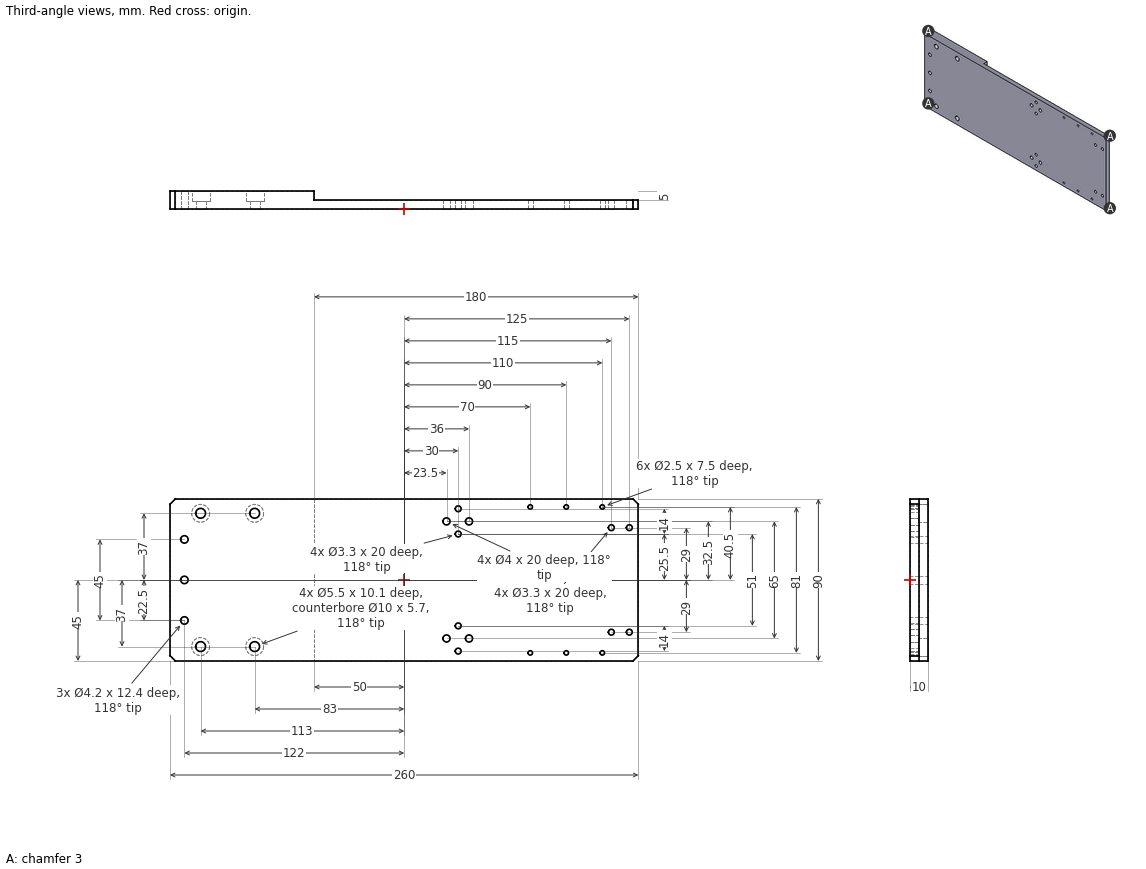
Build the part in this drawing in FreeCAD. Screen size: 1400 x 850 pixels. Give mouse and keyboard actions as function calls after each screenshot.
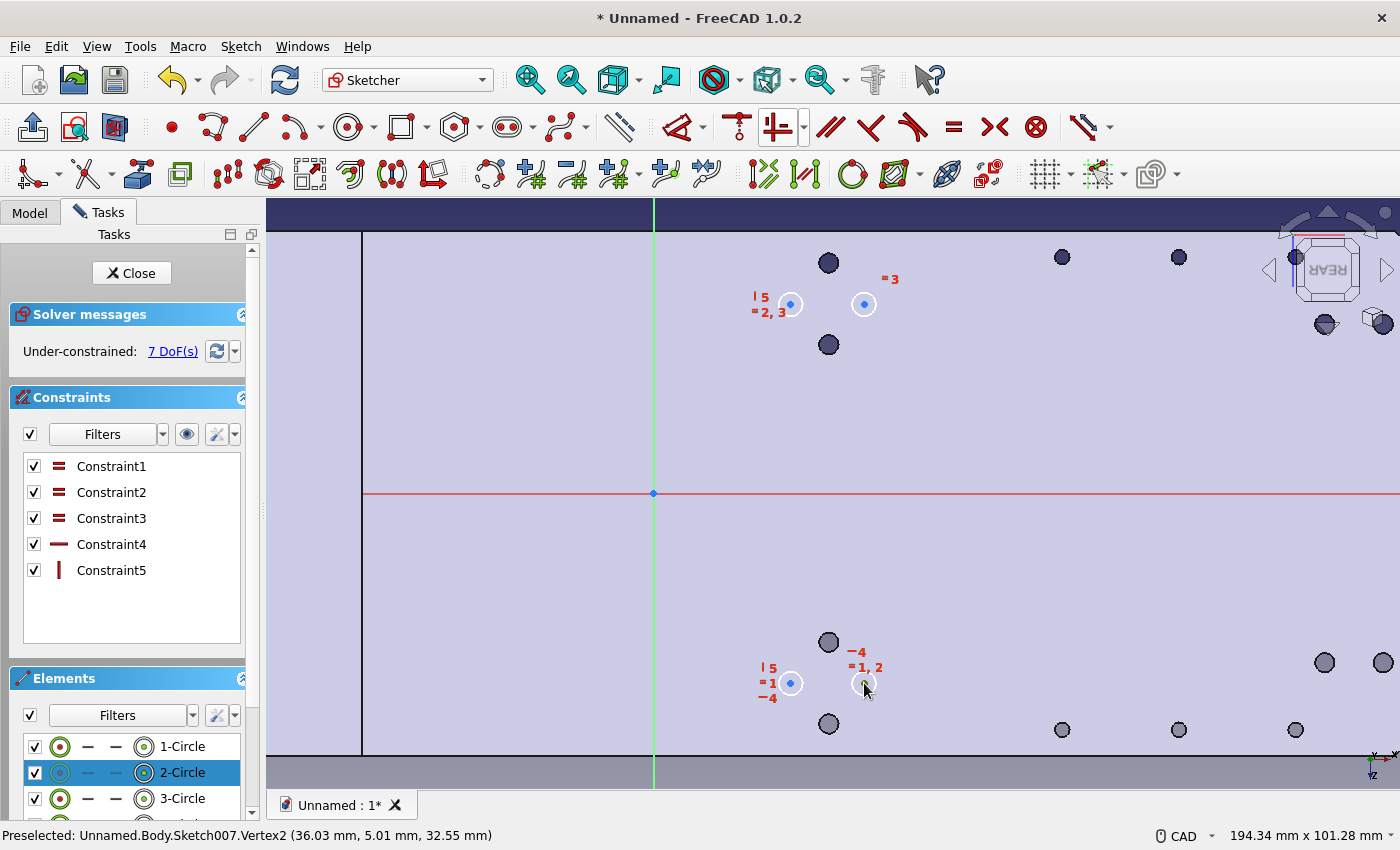
click(864, 304)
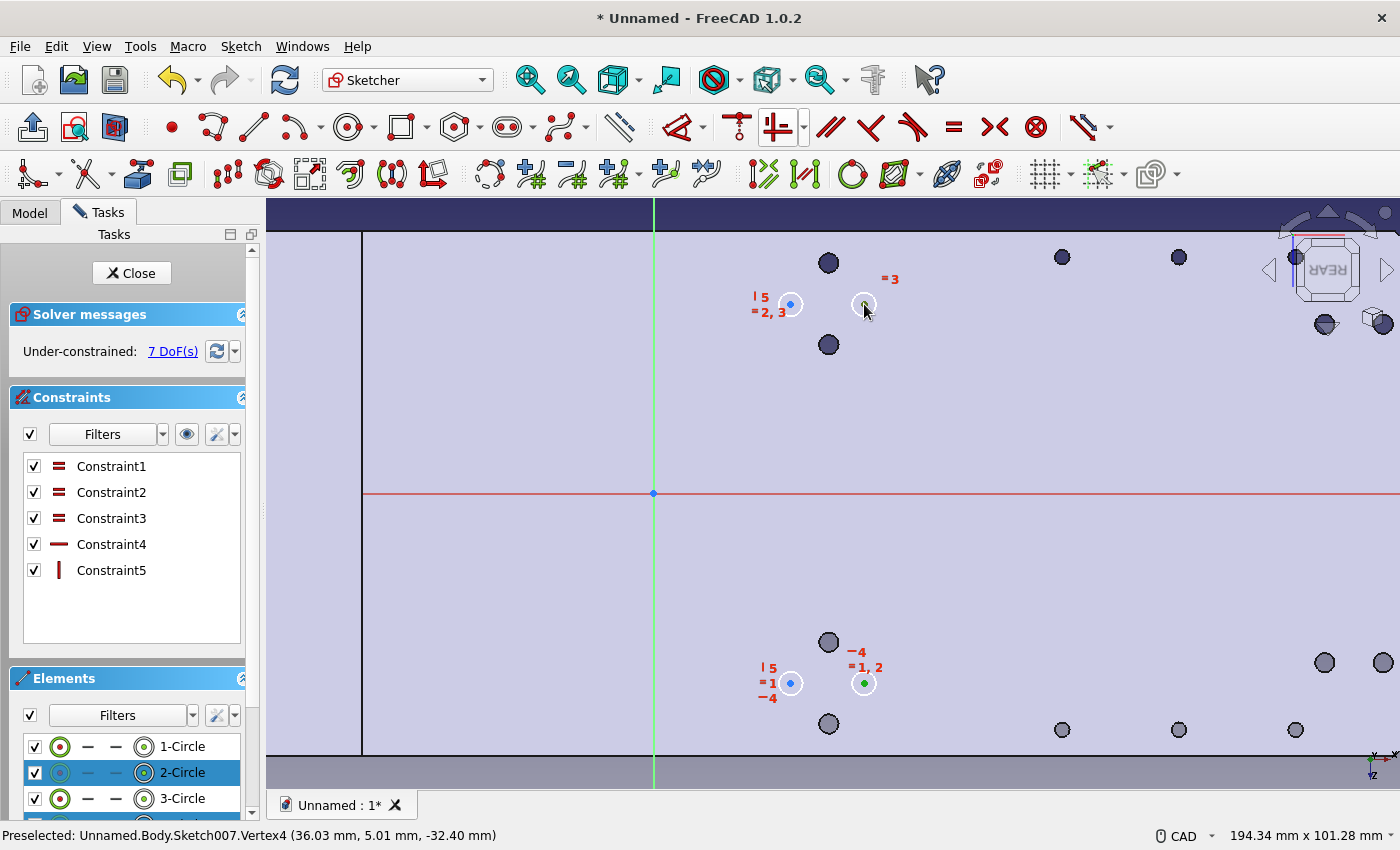
click(804, 128)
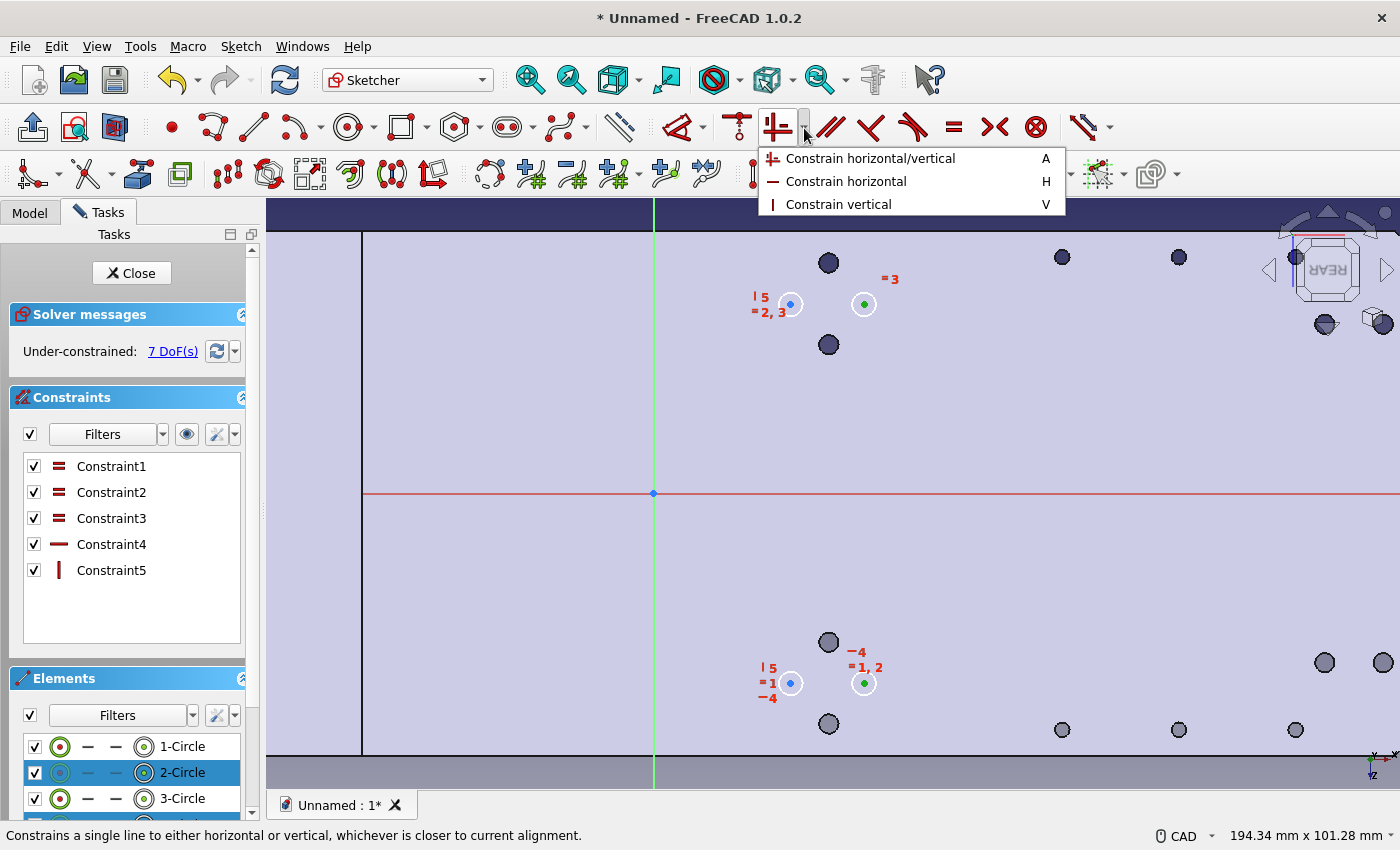
click(912, 204)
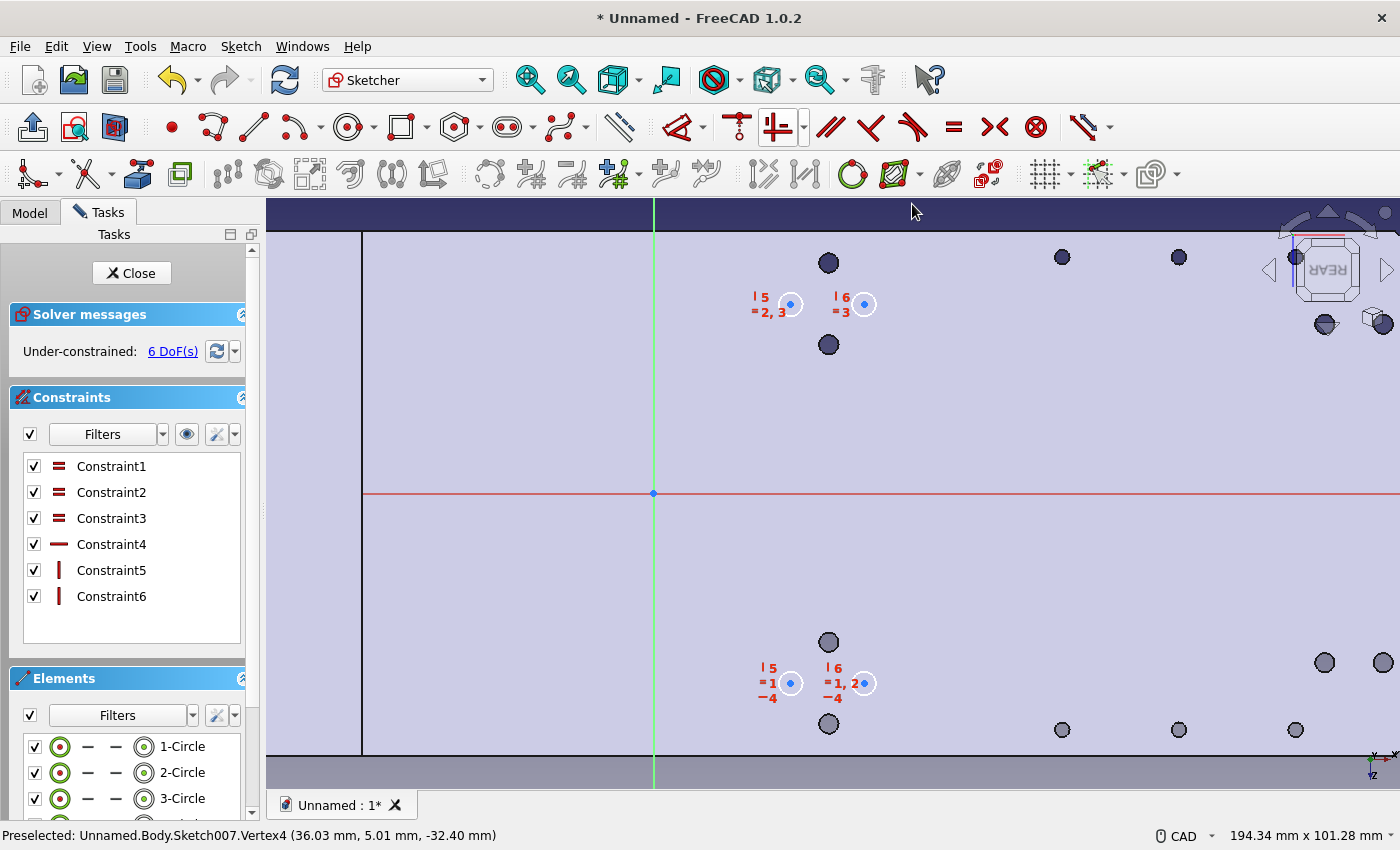
click(791, 304)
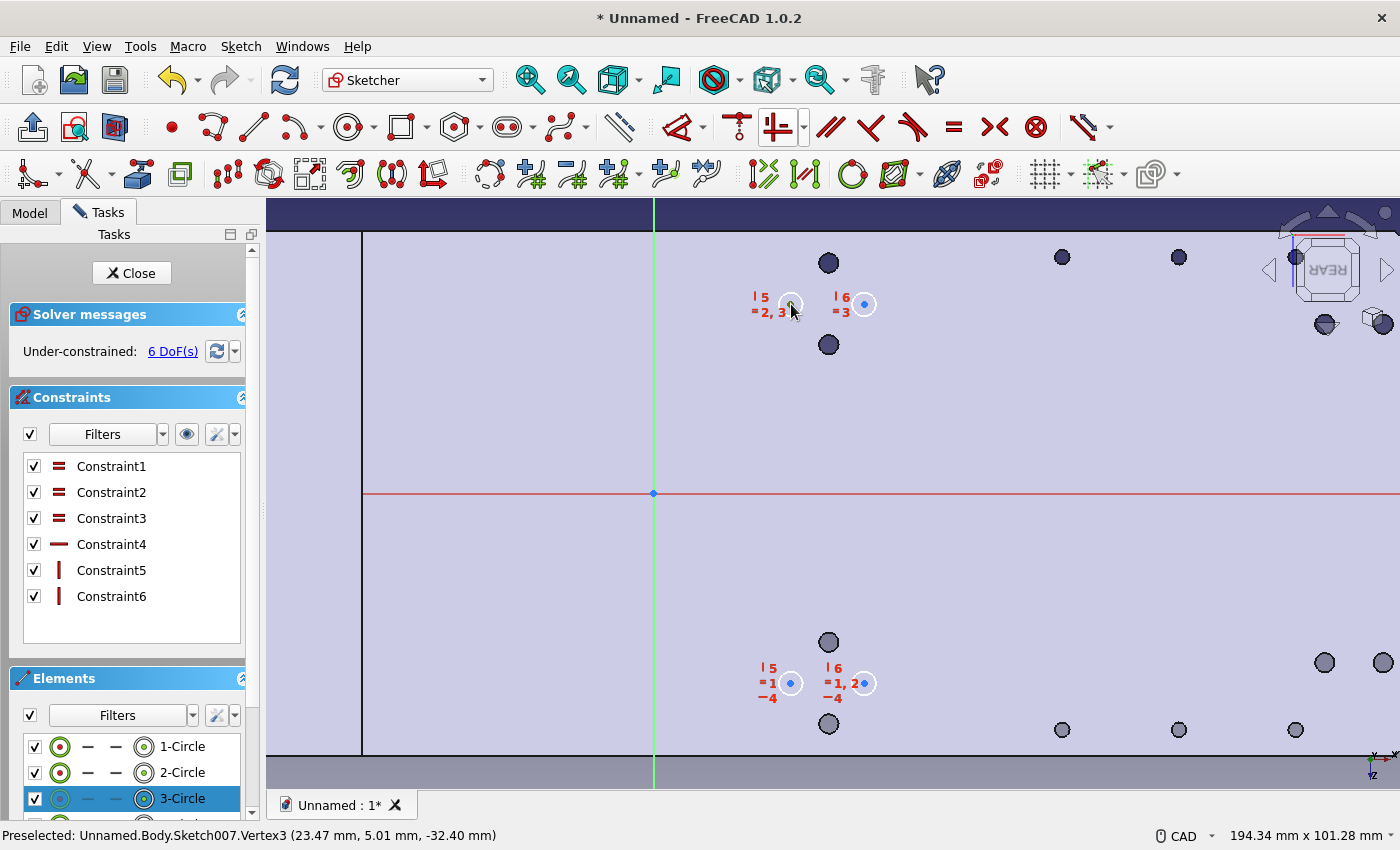
click(864, 304)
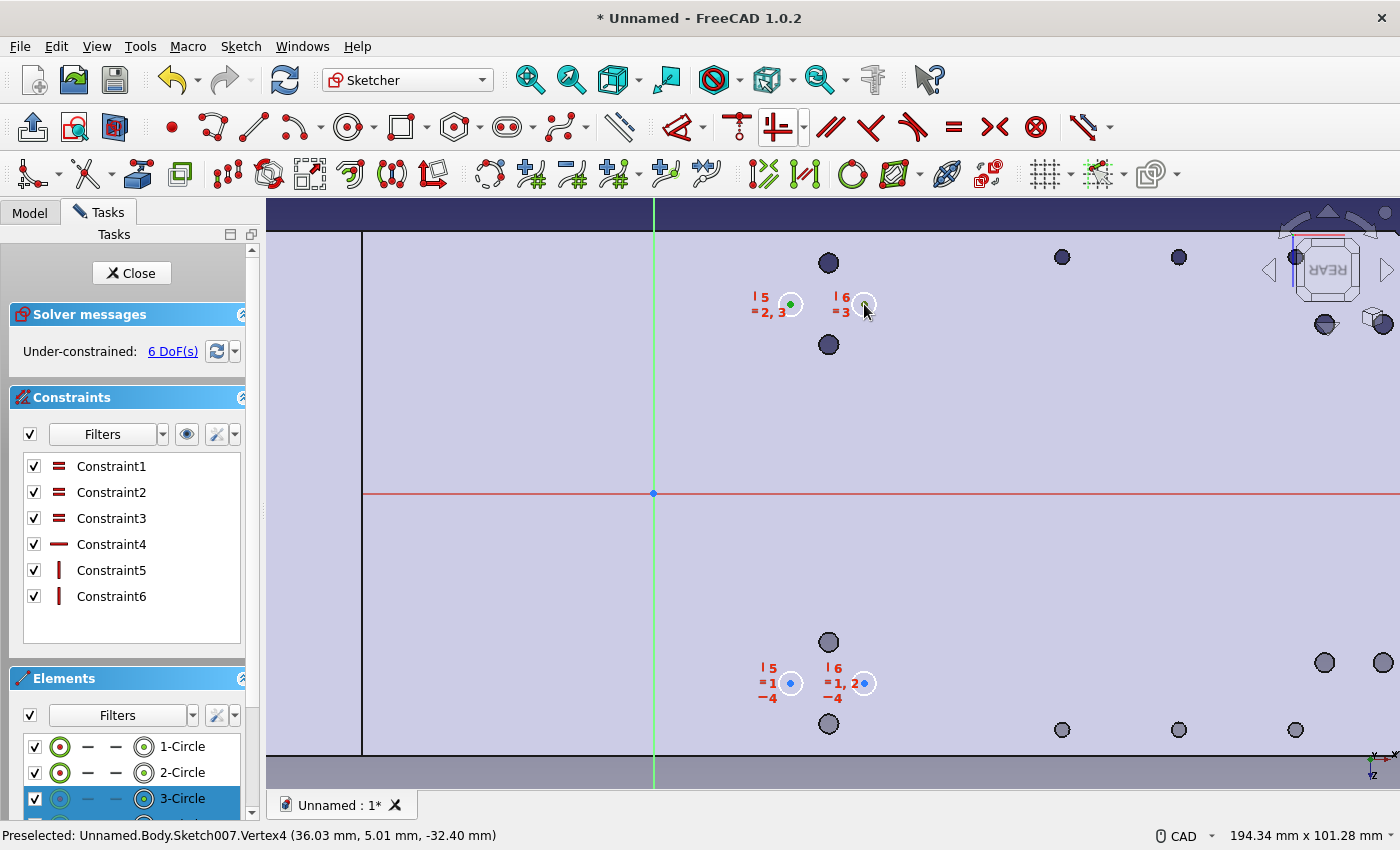
key(h)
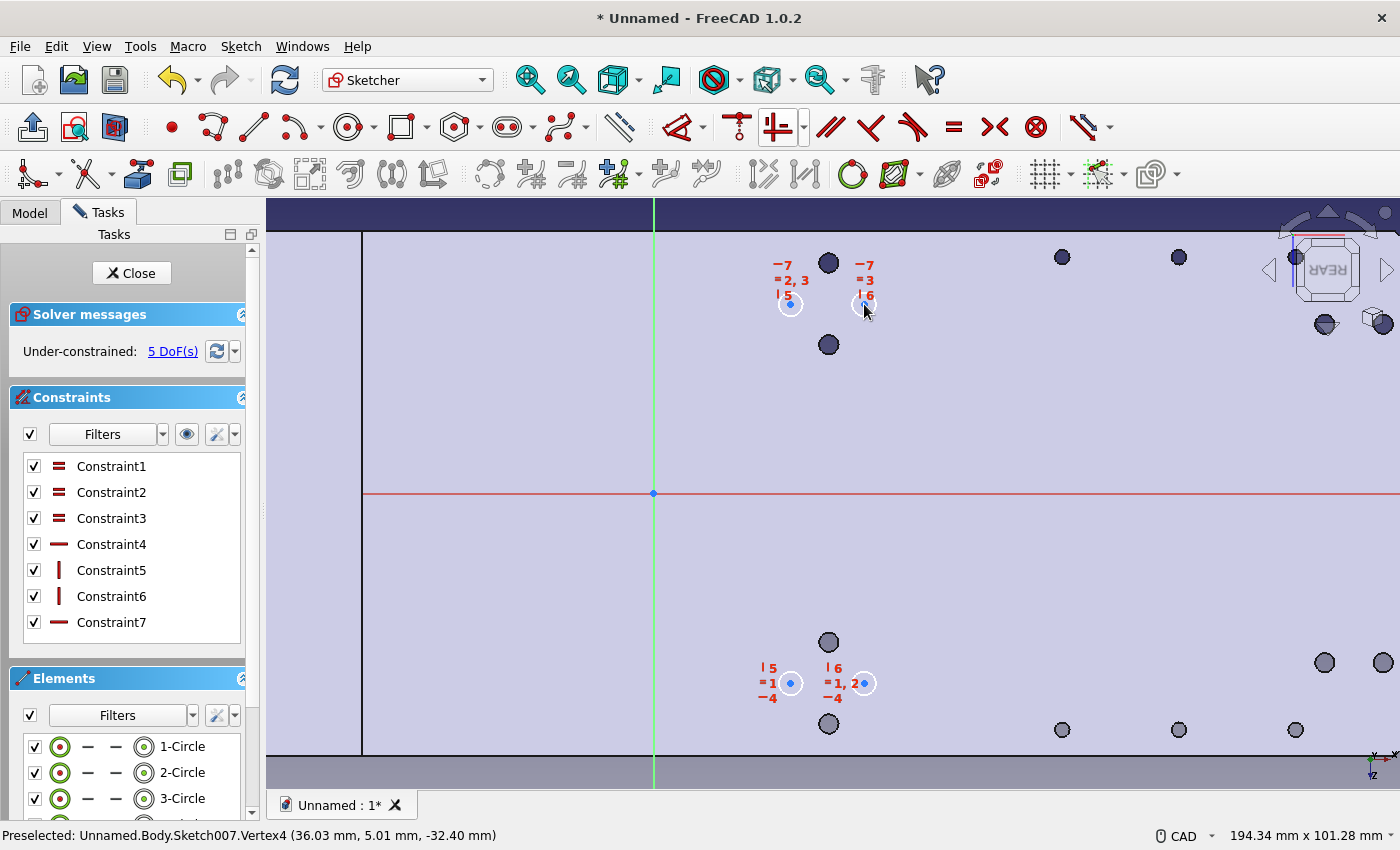
click(676, 128)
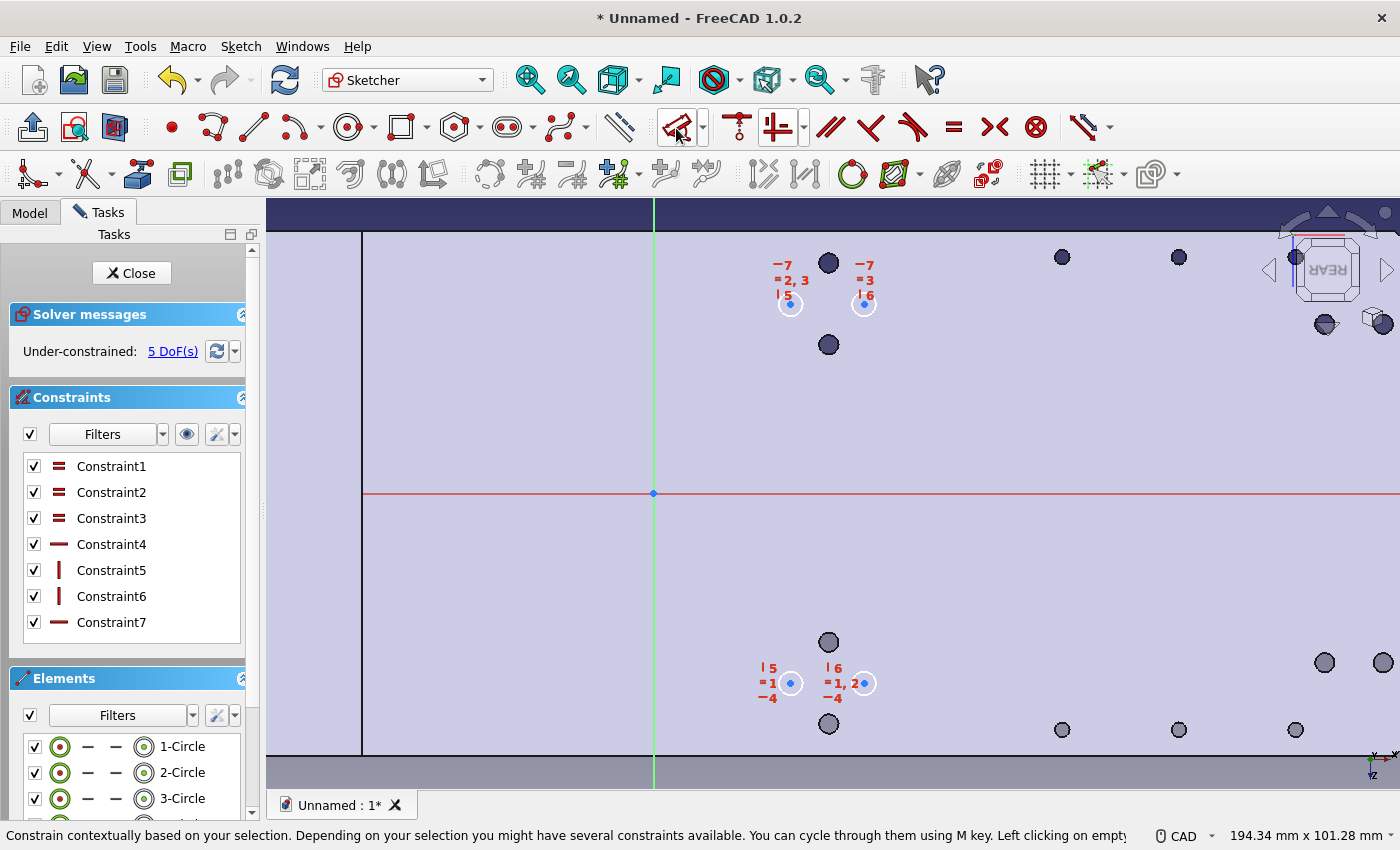
scroll(799, 675, up, 3)